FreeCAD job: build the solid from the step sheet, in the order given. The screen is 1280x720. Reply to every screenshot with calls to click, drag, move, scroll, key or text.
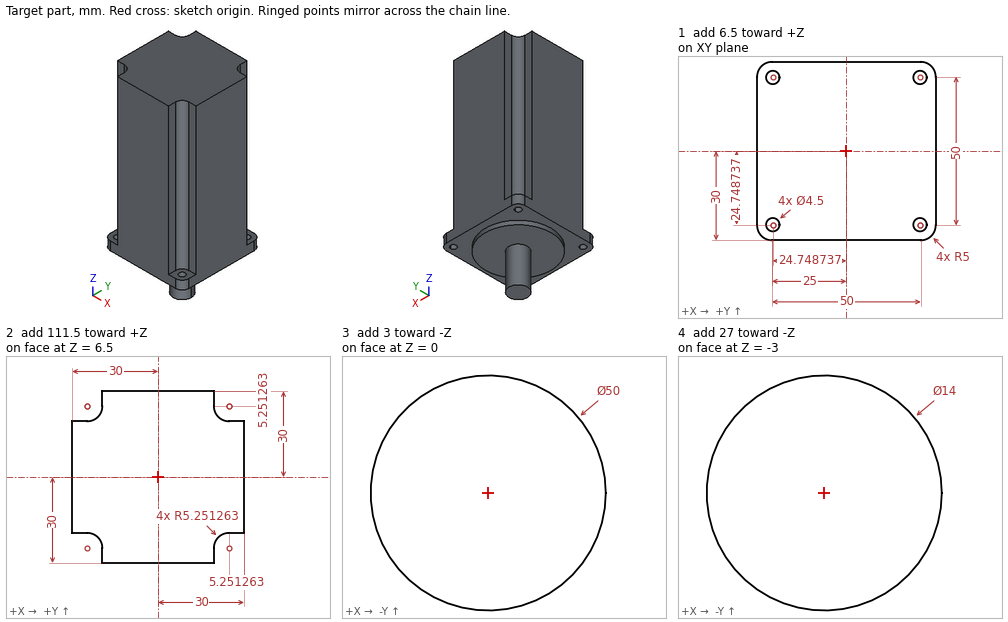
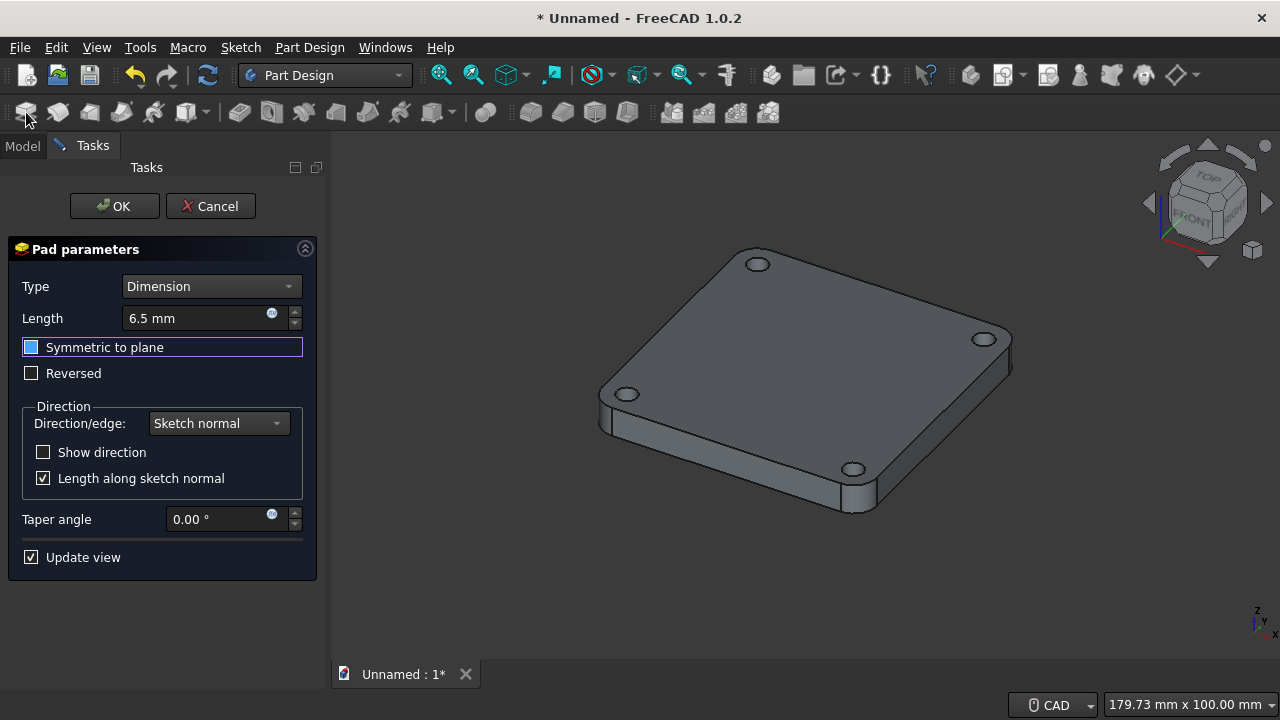
click(115, 206)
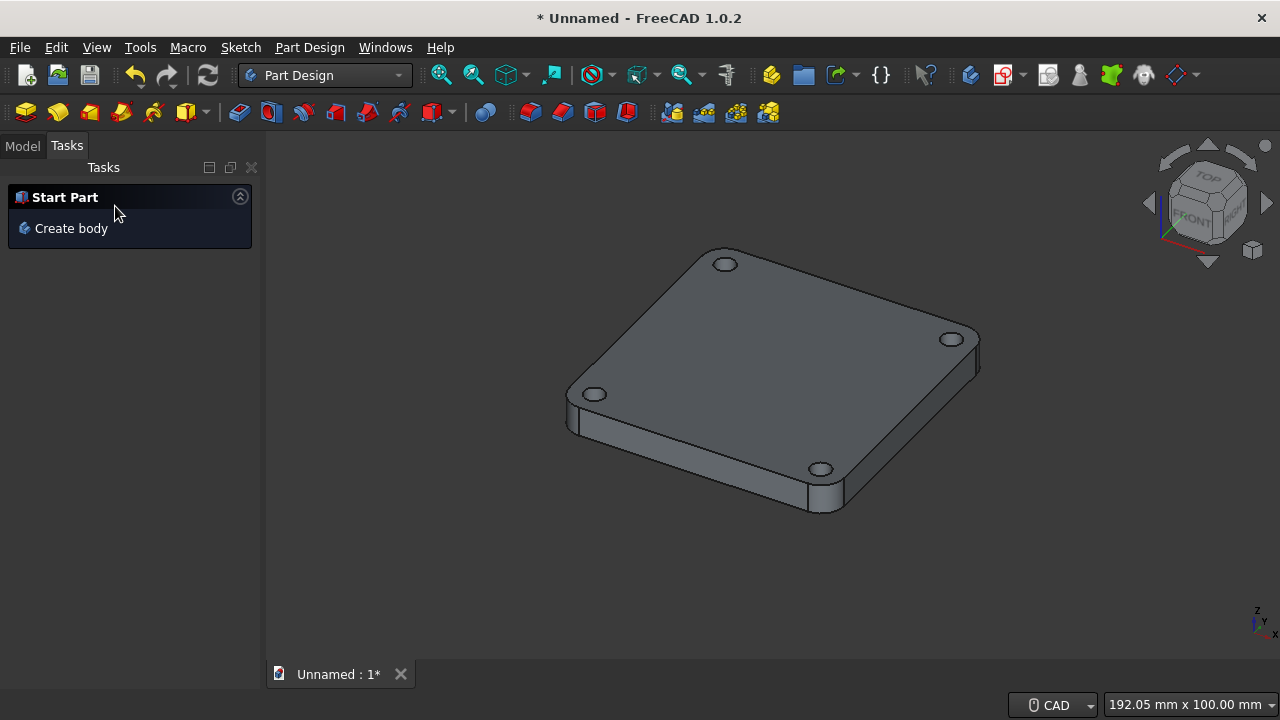
click(773, 366)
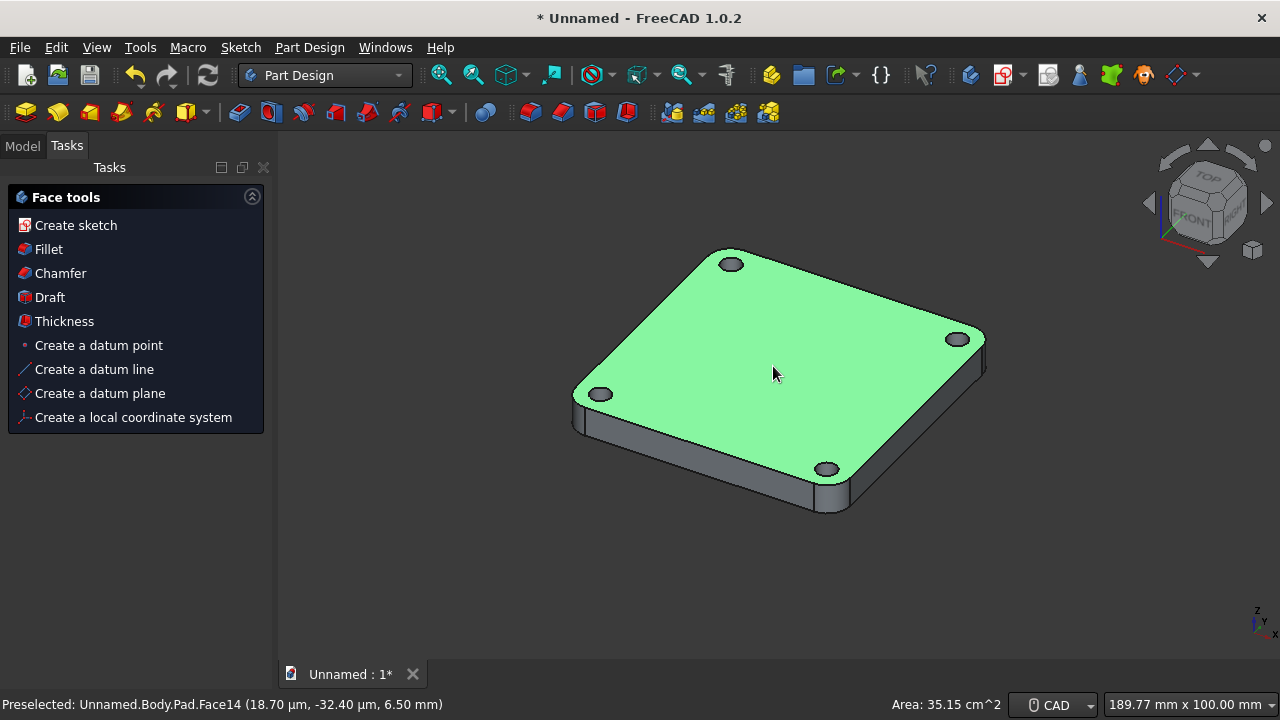
click(1004, 76)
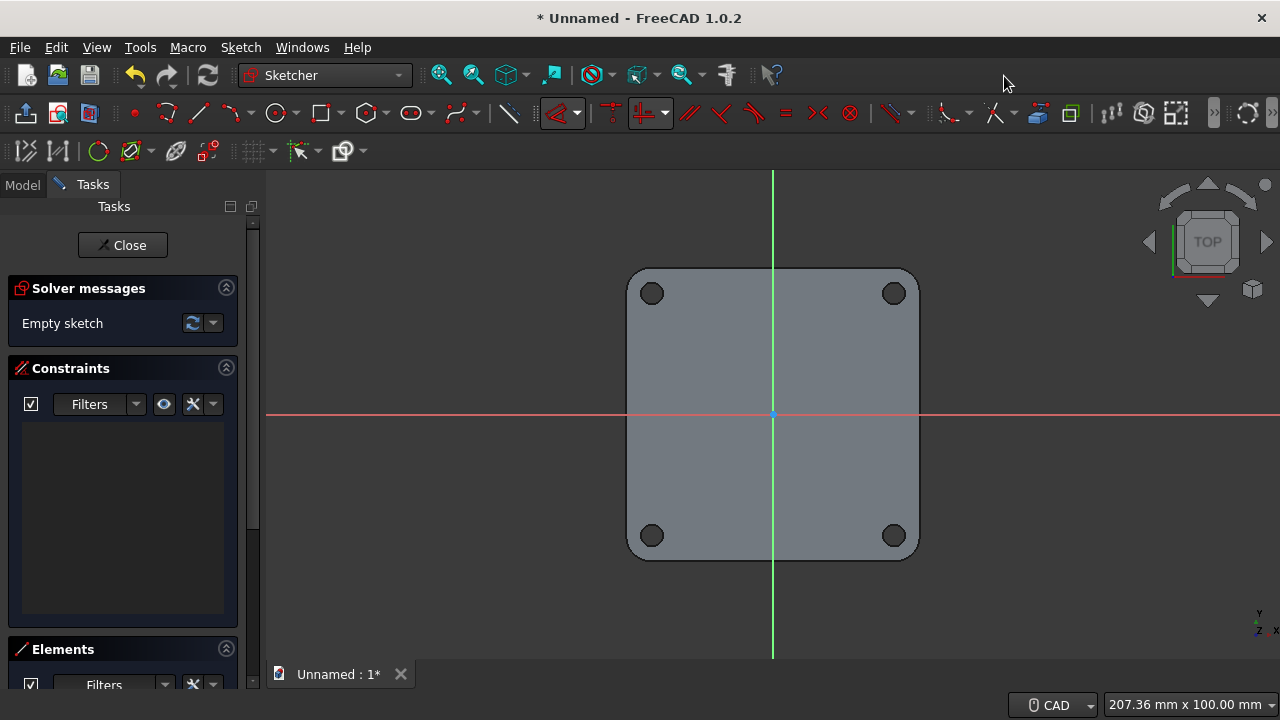
key(g)
key(m)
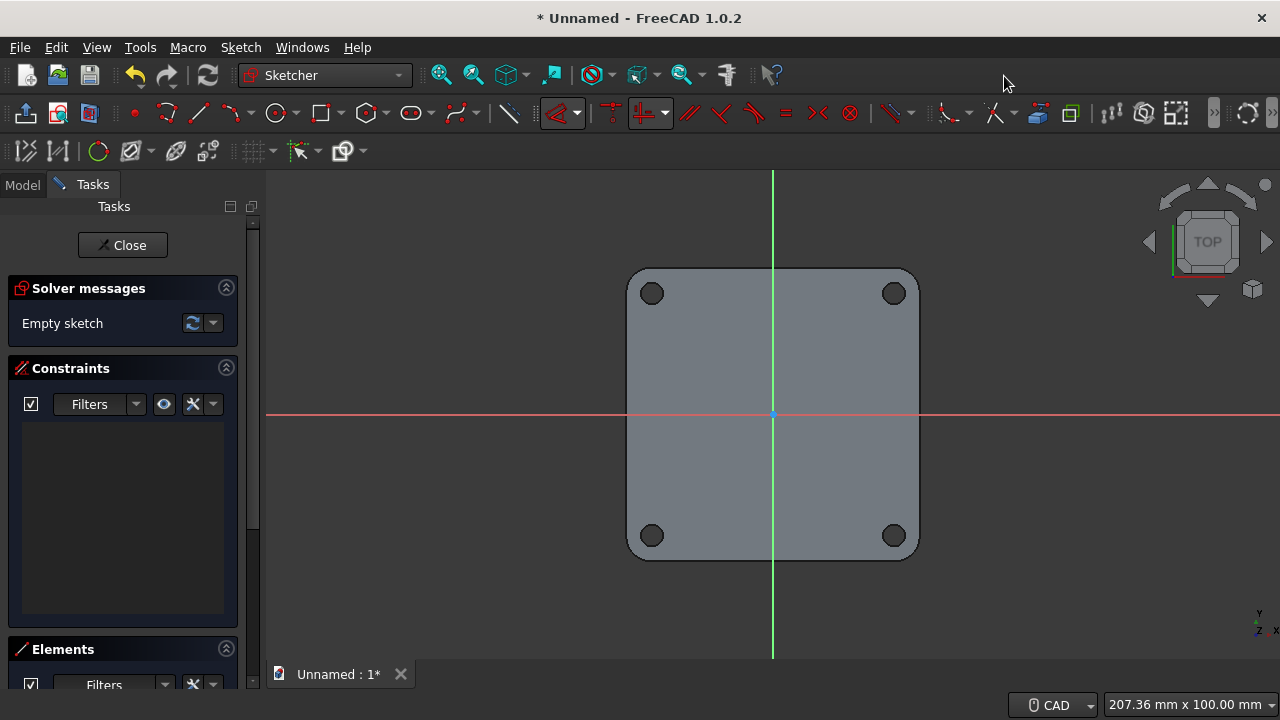
click(894, 510)
click(920, 510)
click(920, 319)
click(894, 319)
right_click(894, 319)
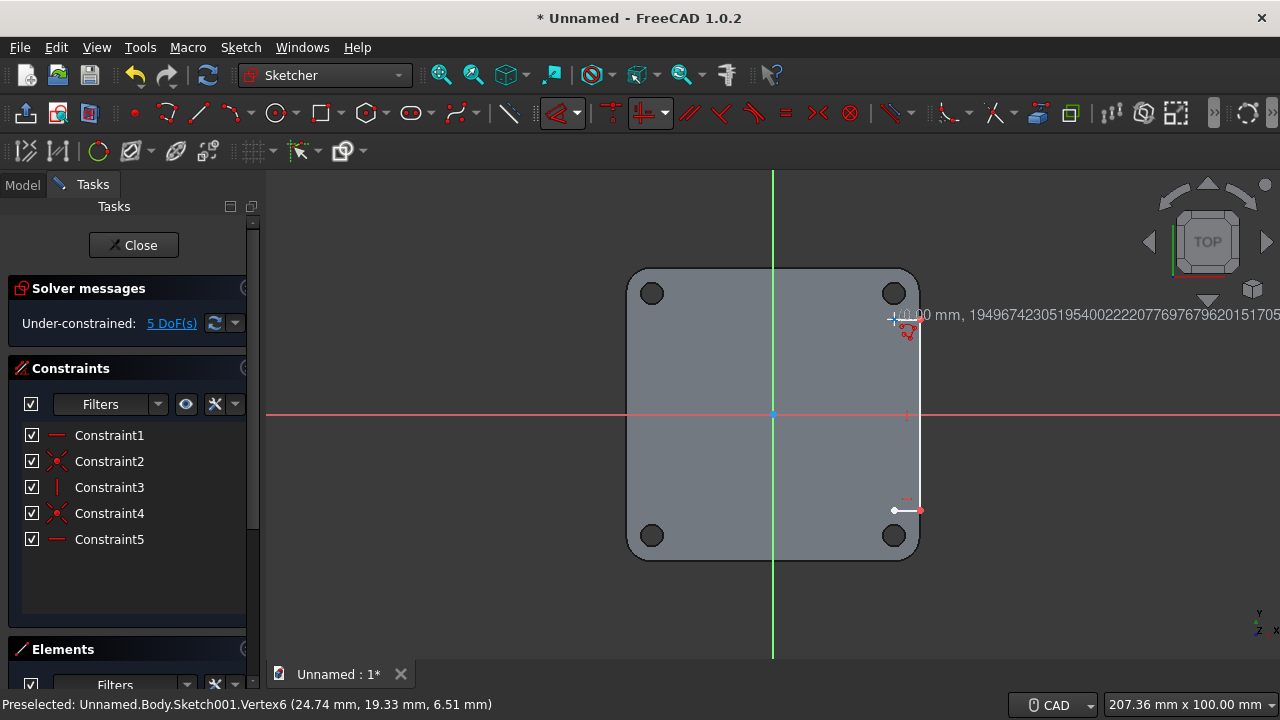
click(868, 293)
click(868, 268)
click(678, 268)
click(678, 293)
right_click(678, 293)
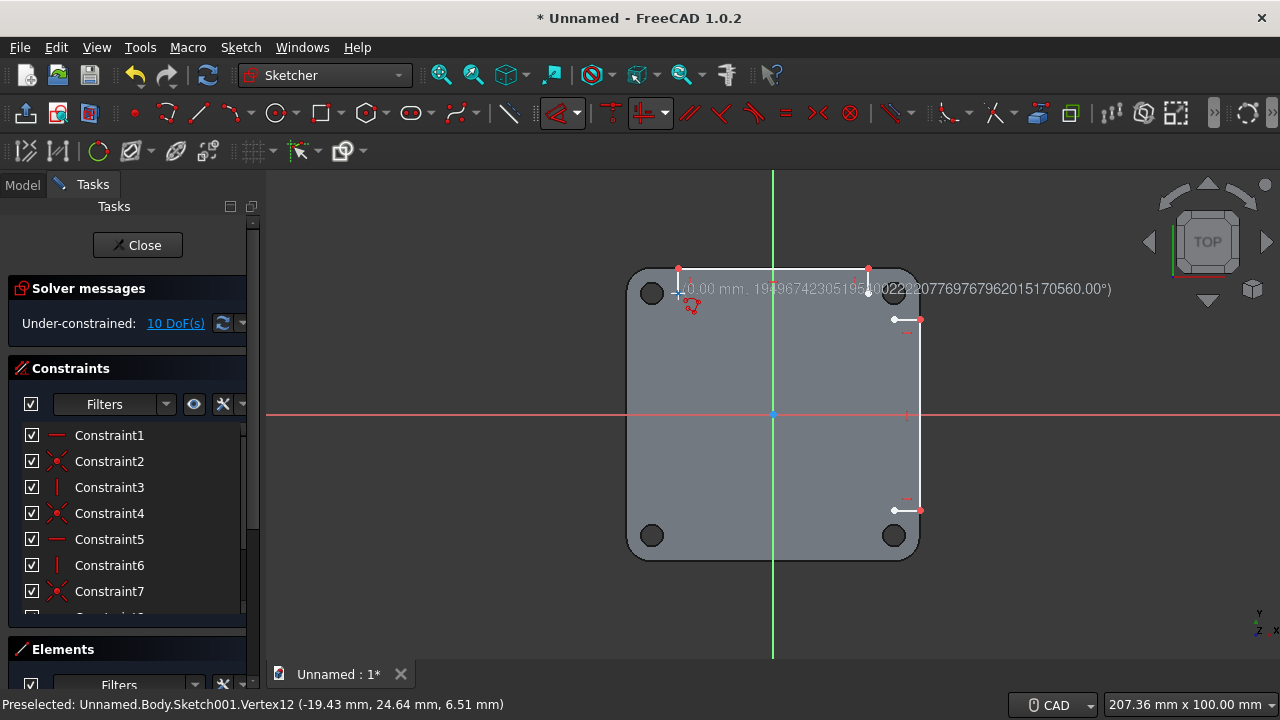
click(652, 319)
click(626, 319)
click(626, 510)
click(652, 510)
right_click(652, 510)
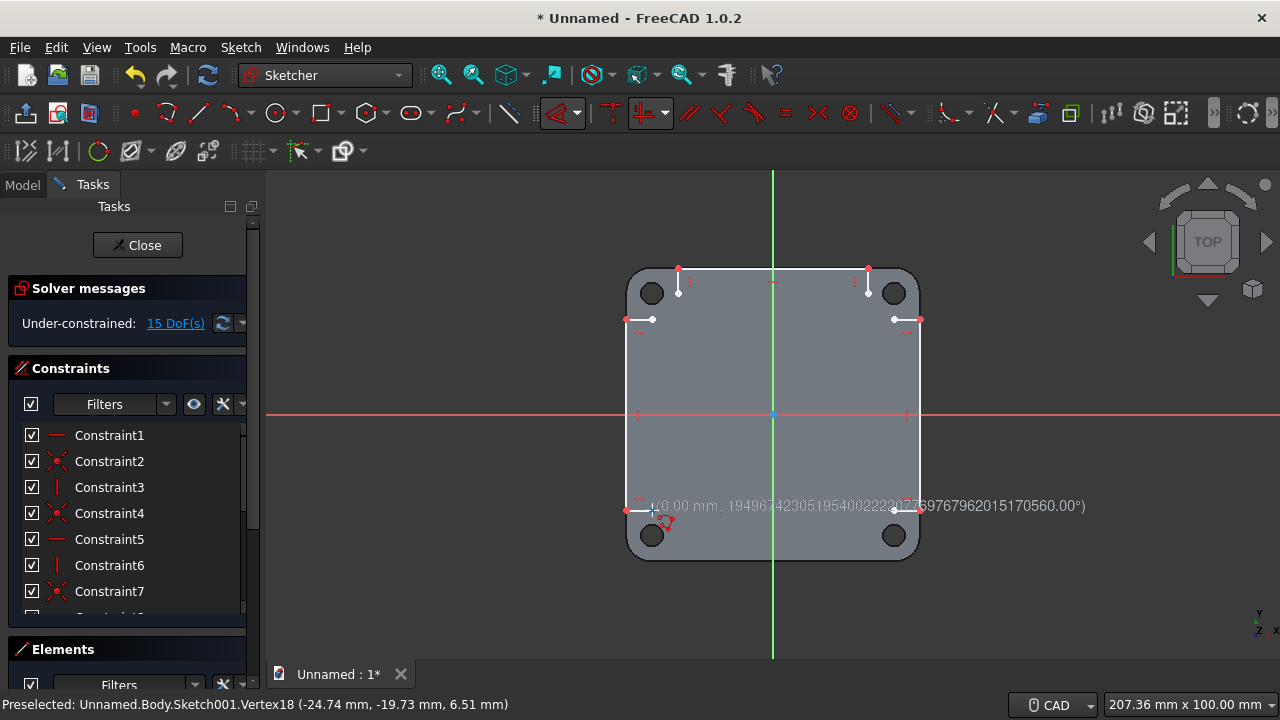
click(678, 536)
click(678, 561)
click(868, 561)
click(868, 536)
right_click(868, 536)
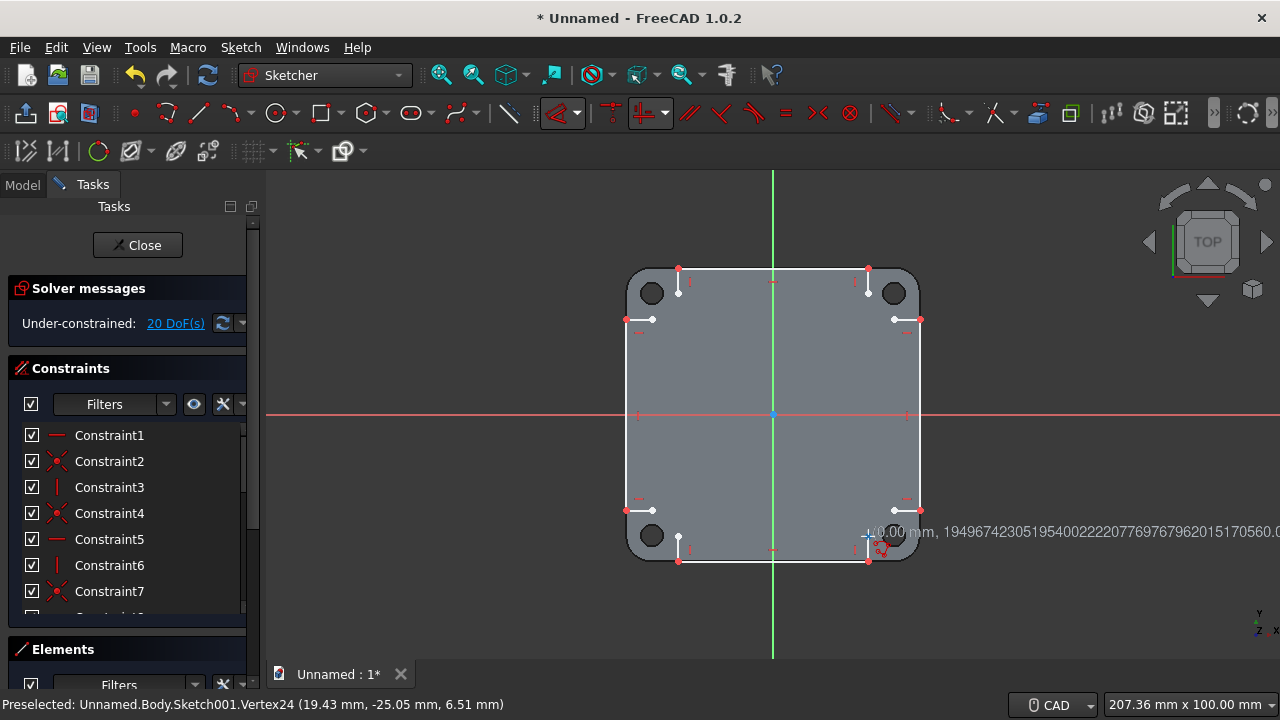
key(g)
key(3)
key(a)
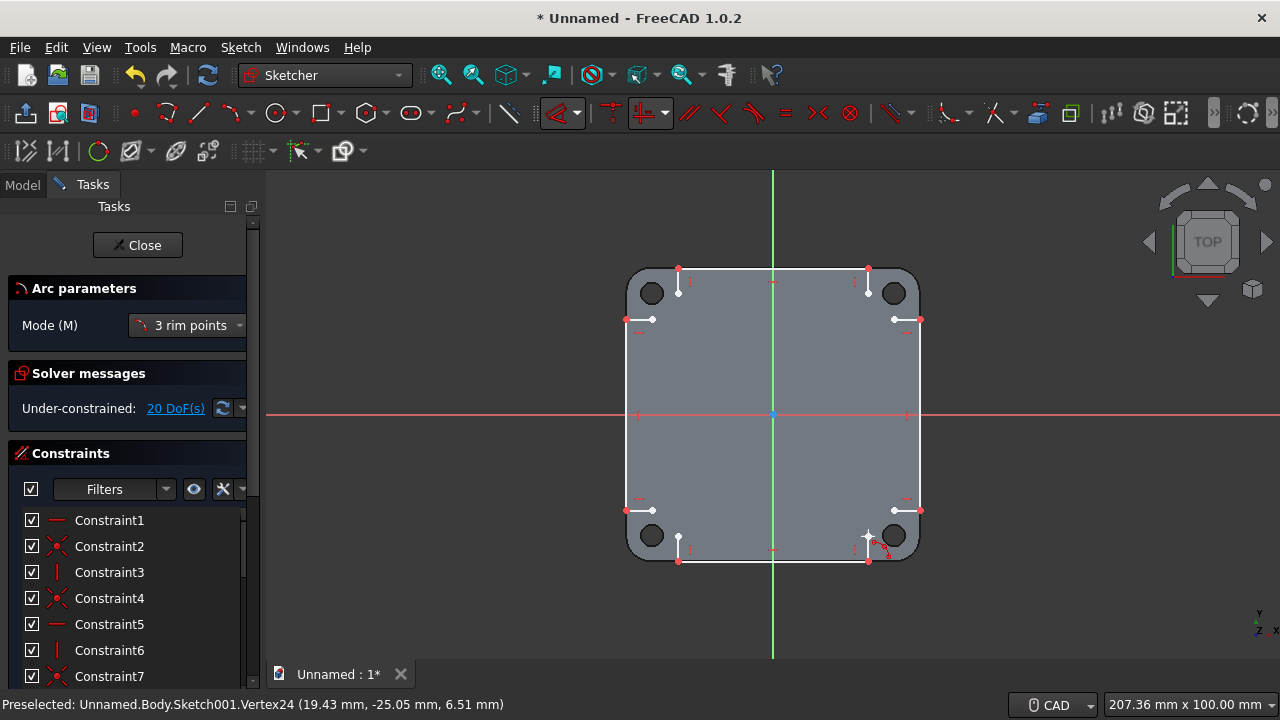
scroll(894, 319, up, 2)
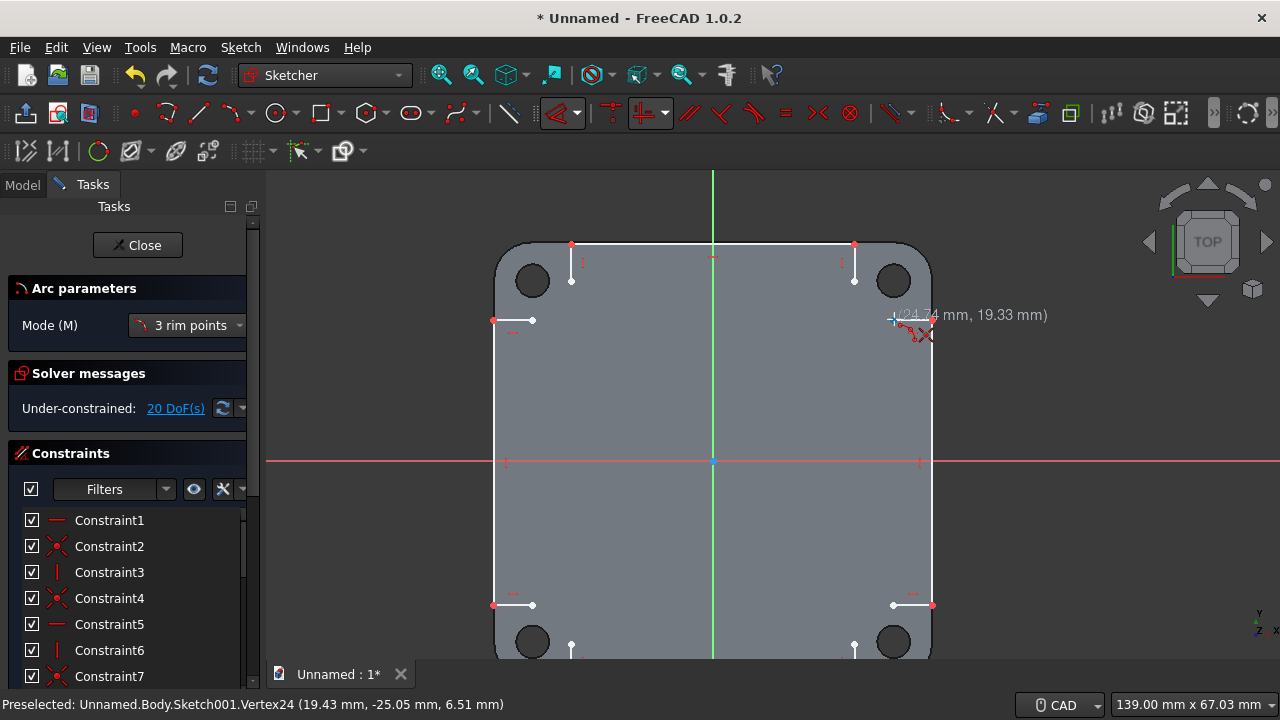
click(894, 320)
click(855, 282)